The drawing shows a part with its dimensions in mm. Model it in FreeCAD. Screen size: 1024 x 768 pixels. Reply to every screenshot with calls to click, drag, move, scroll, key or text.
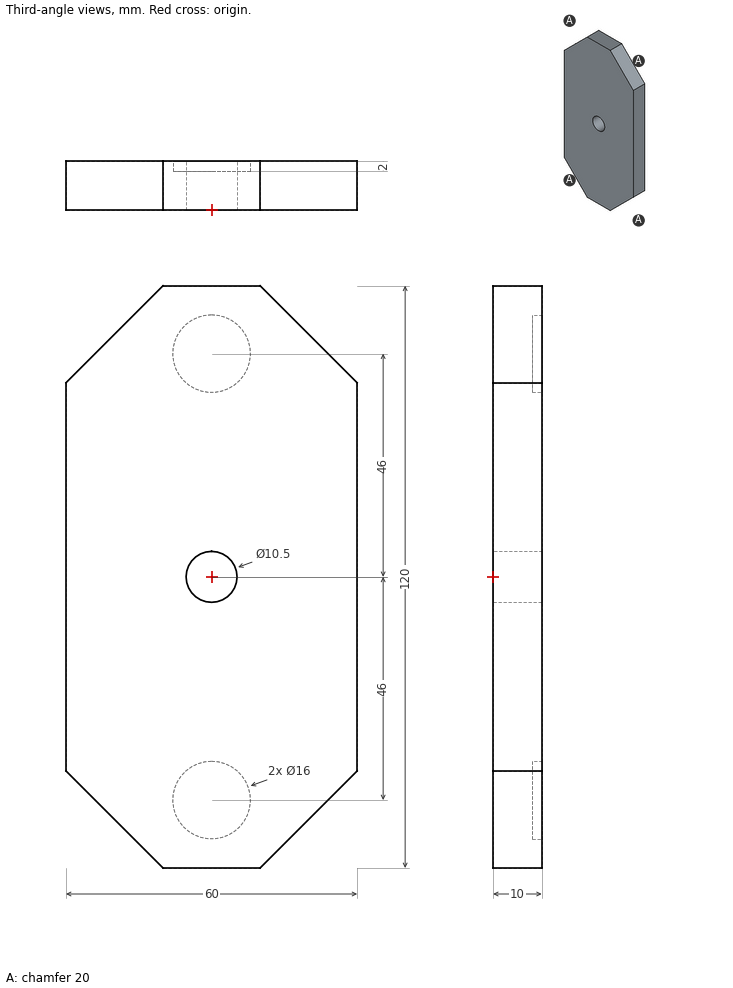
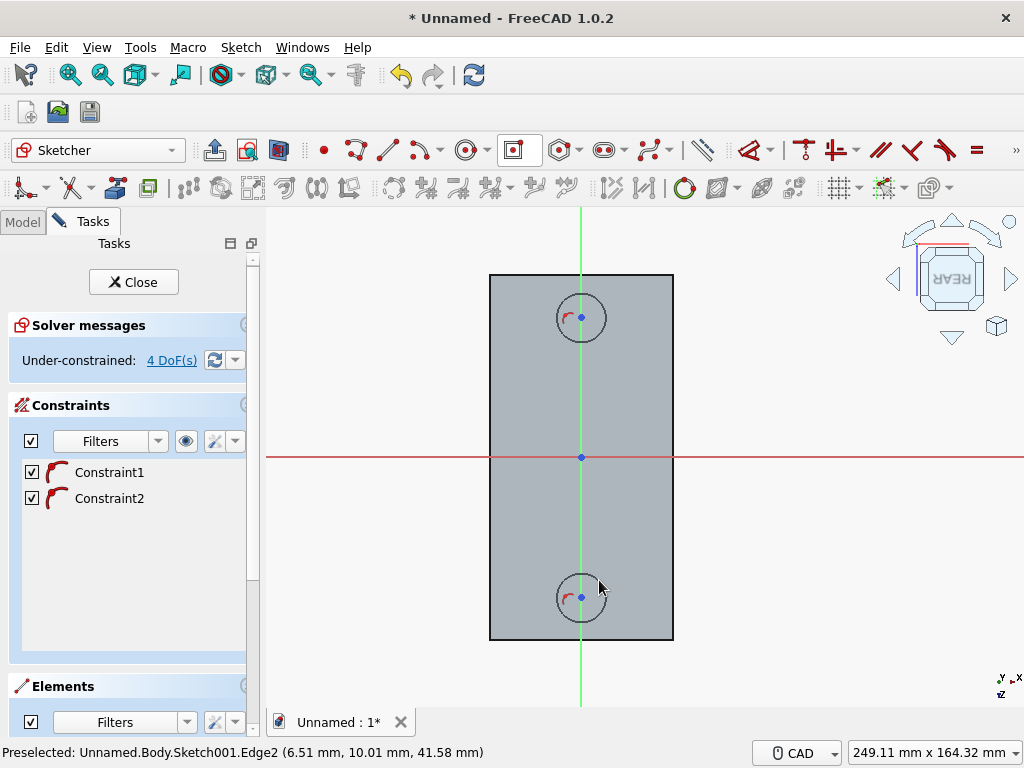
click(599, 301)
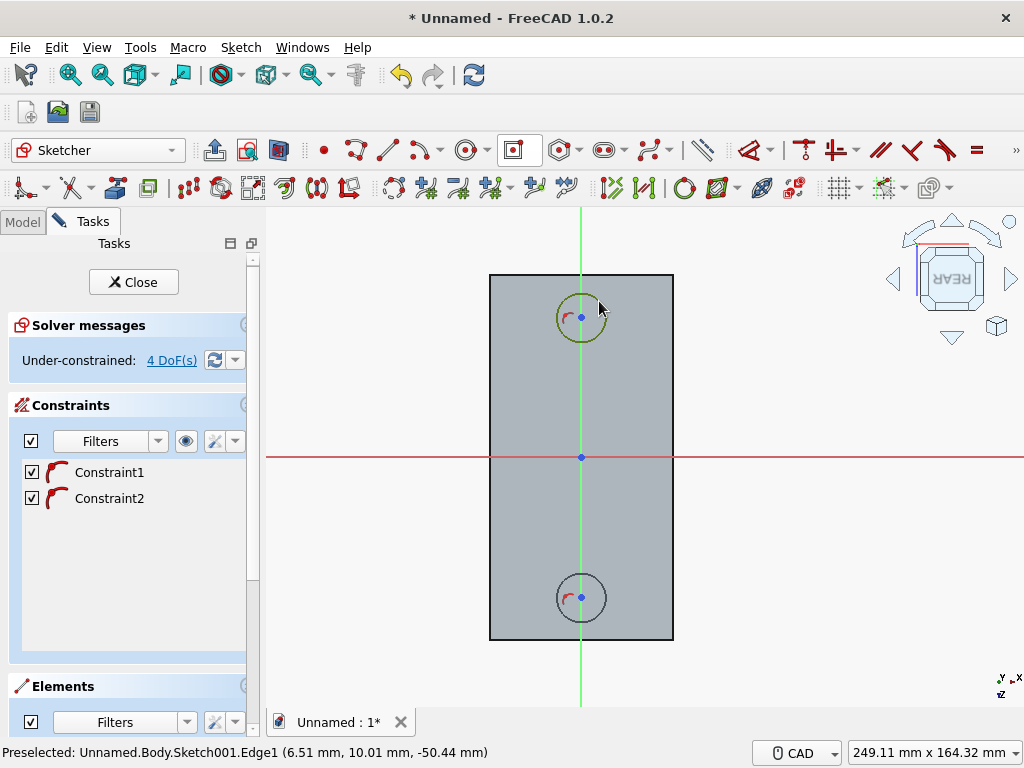
click(599, 581)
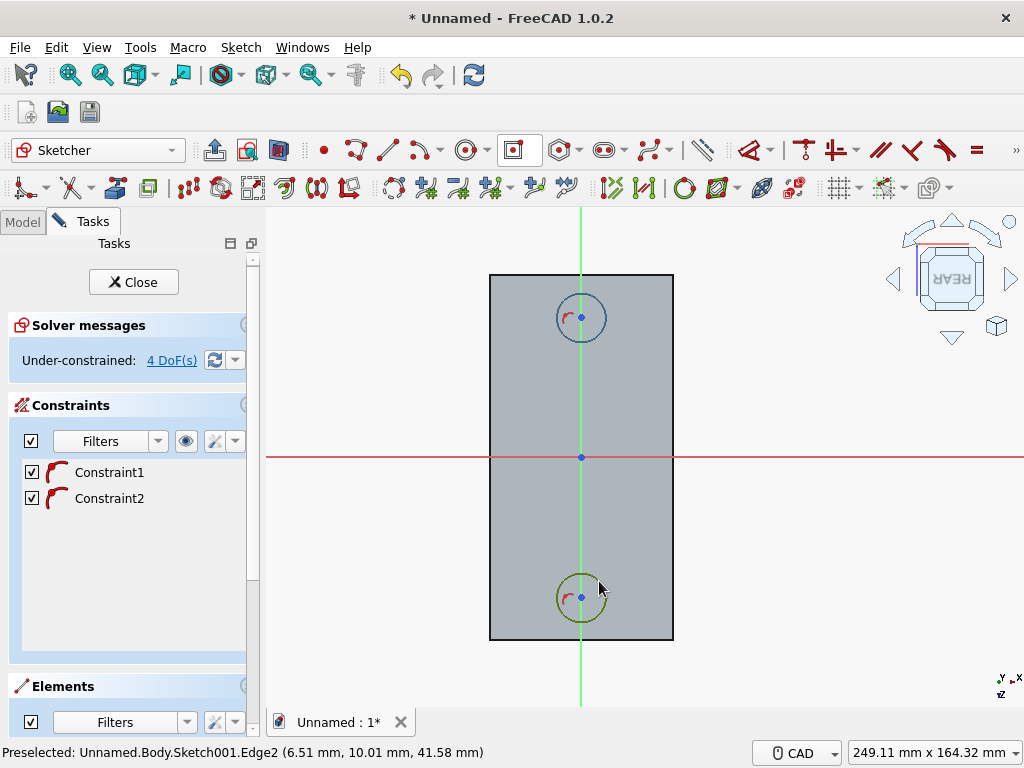
click(978, 150)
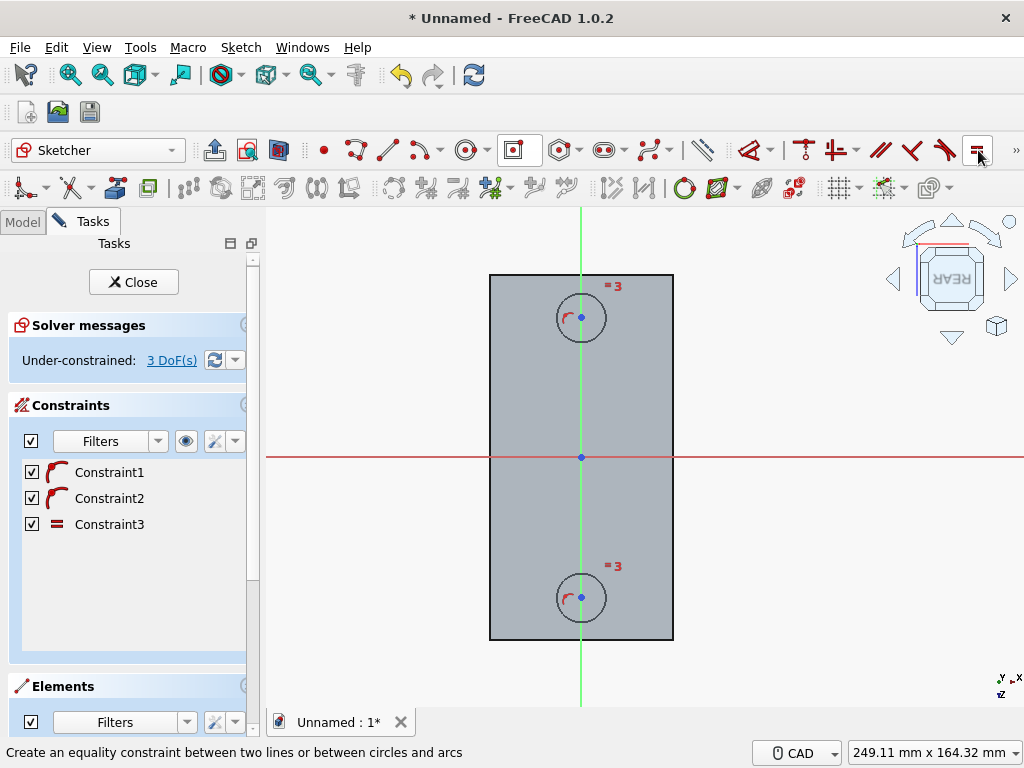
click(750, 150)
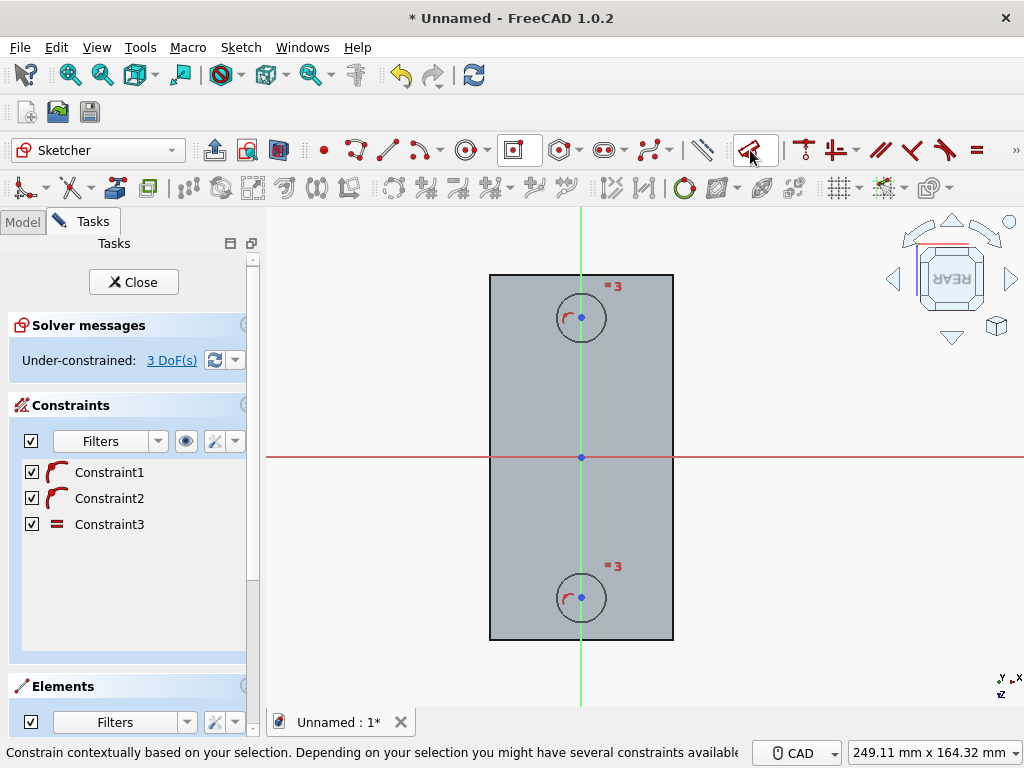
click(599, 301)
click(622, 279)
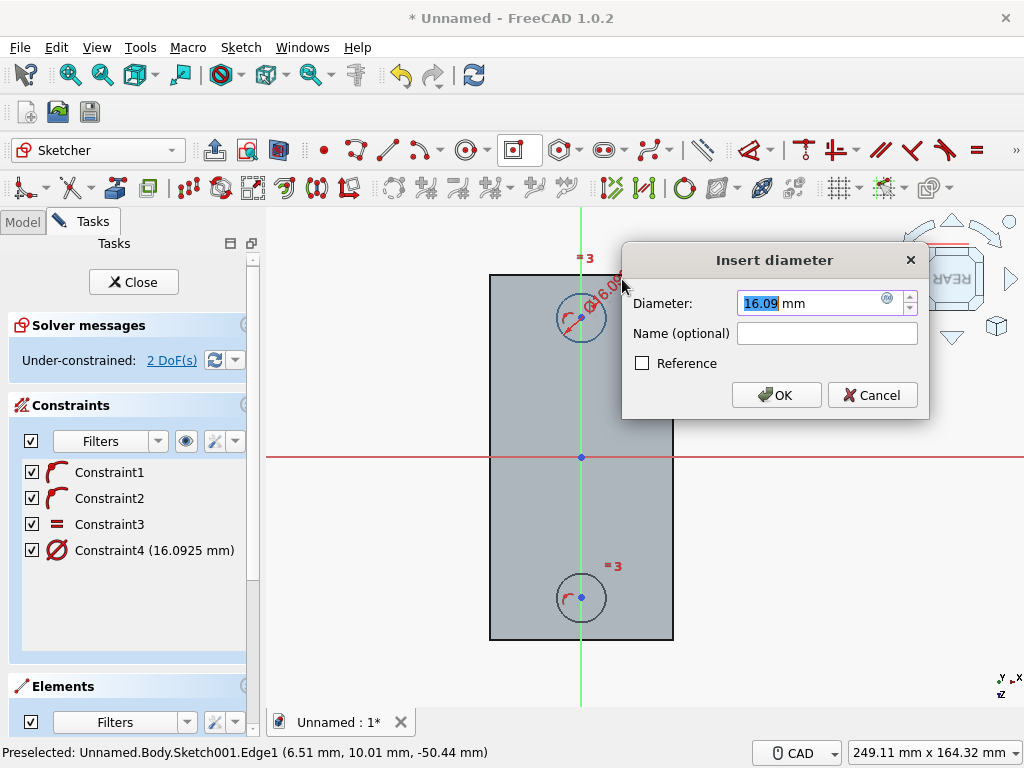
text(16)
key(Return)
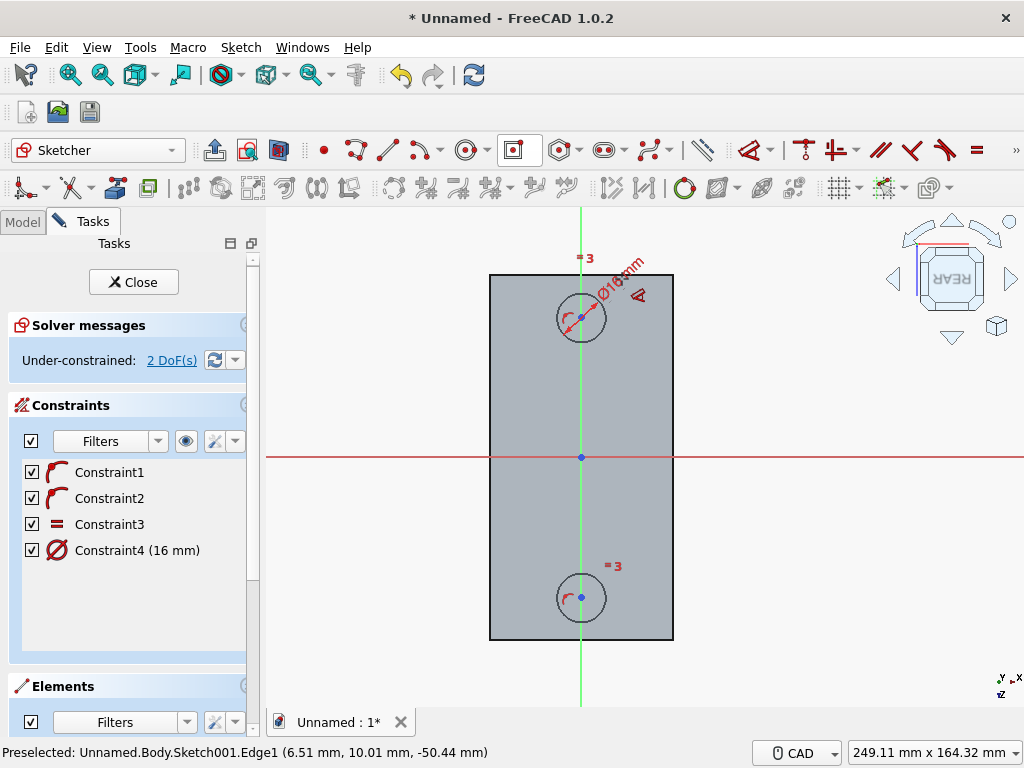
click(581, 318)
click(615, 388)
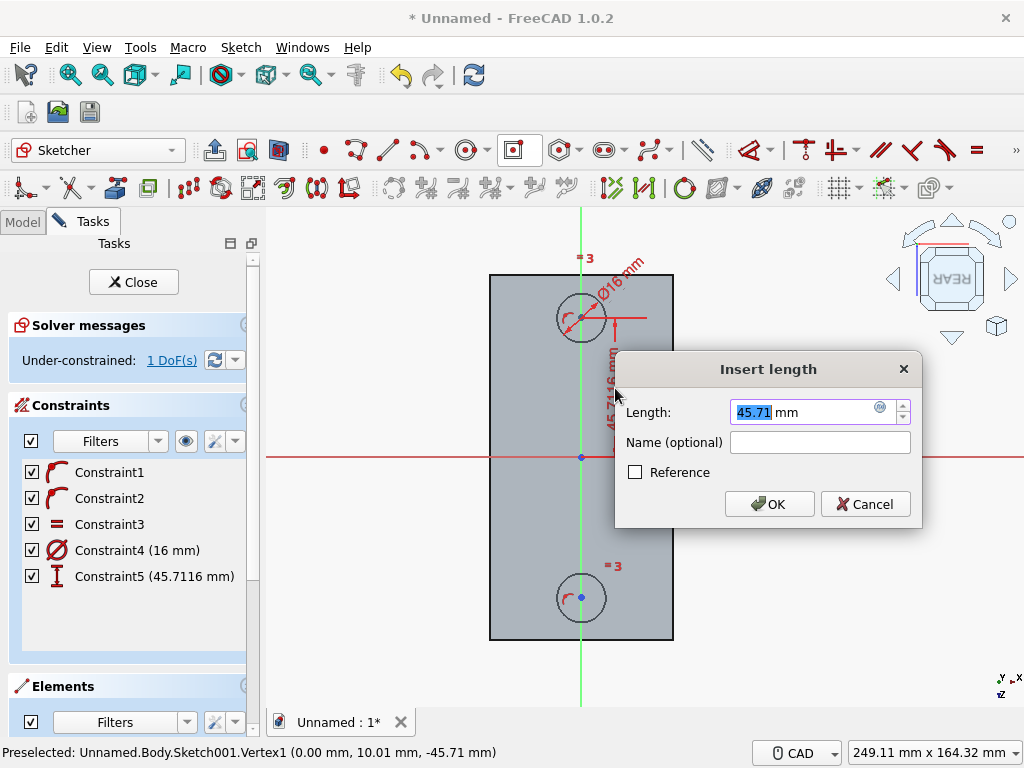
text(46)
key(Return)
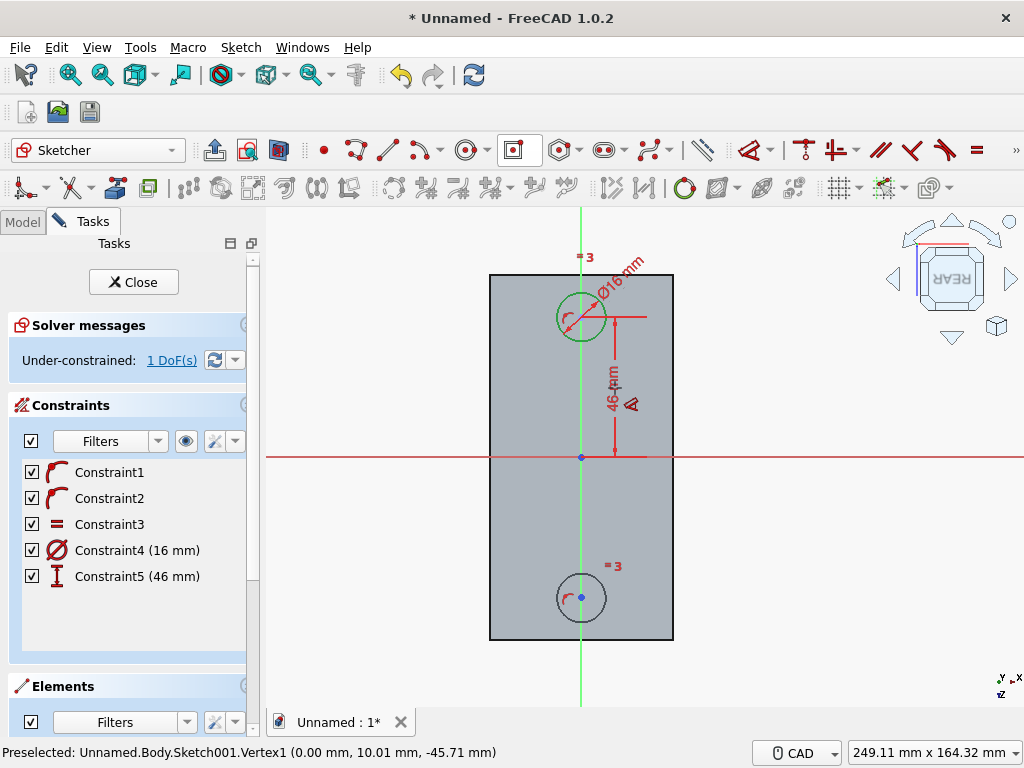
click(581, 598)
click(615, 528)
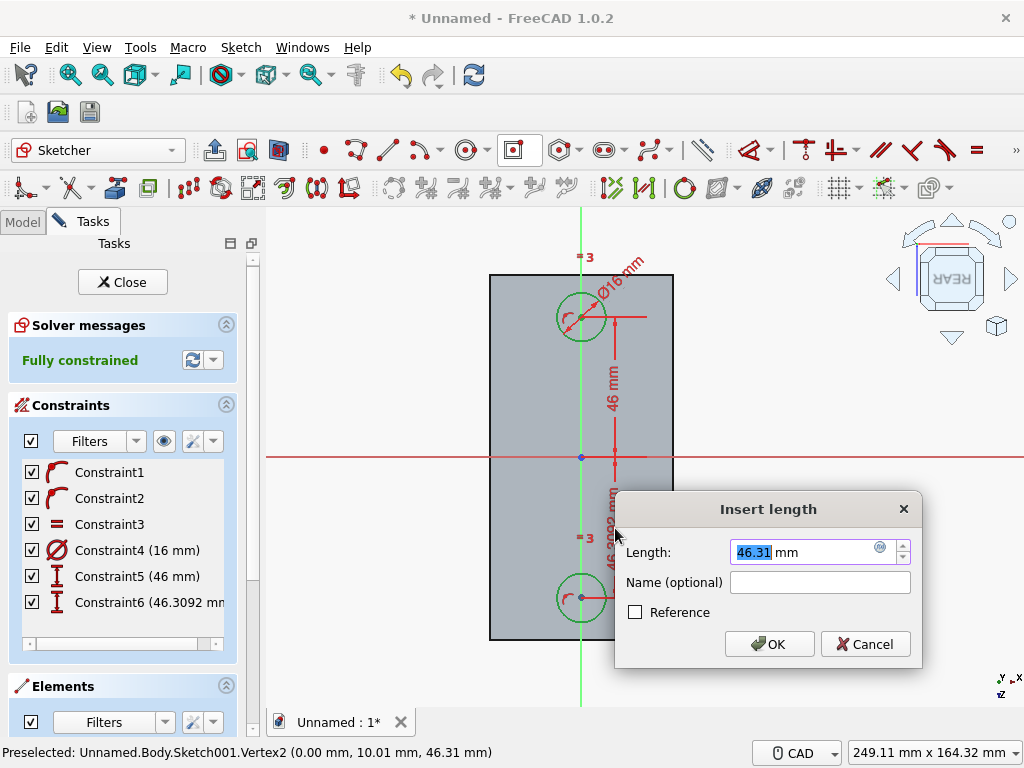
text(46)
key(Return)
key(Escape)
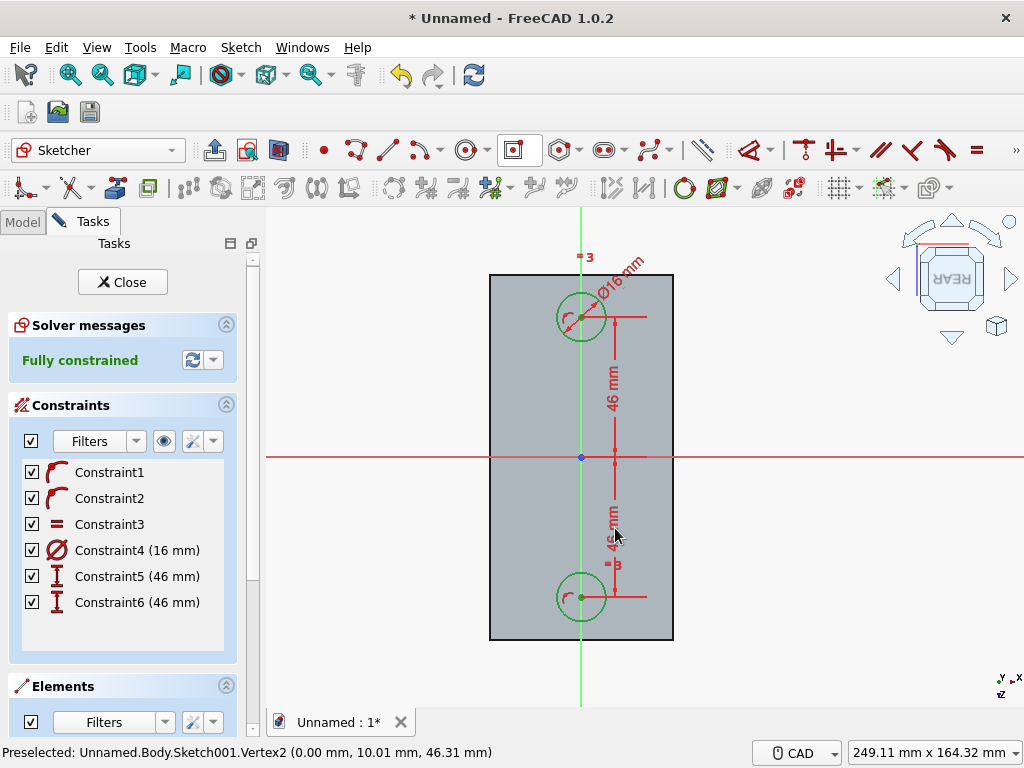
click(123, 282)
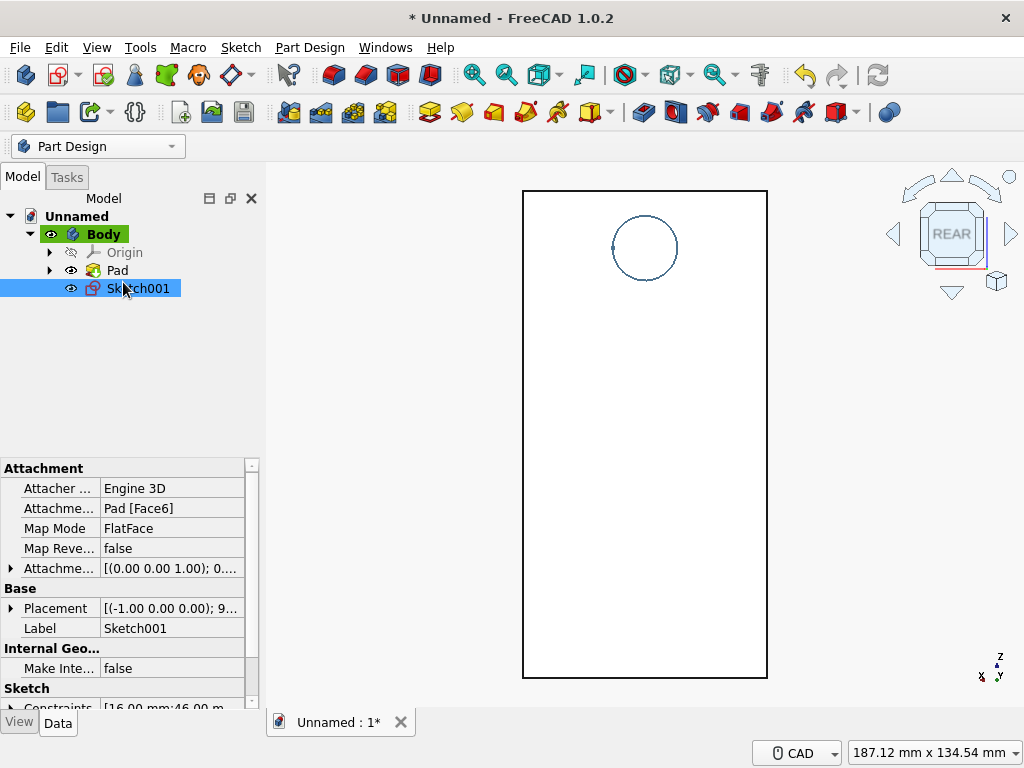
click(644, 112)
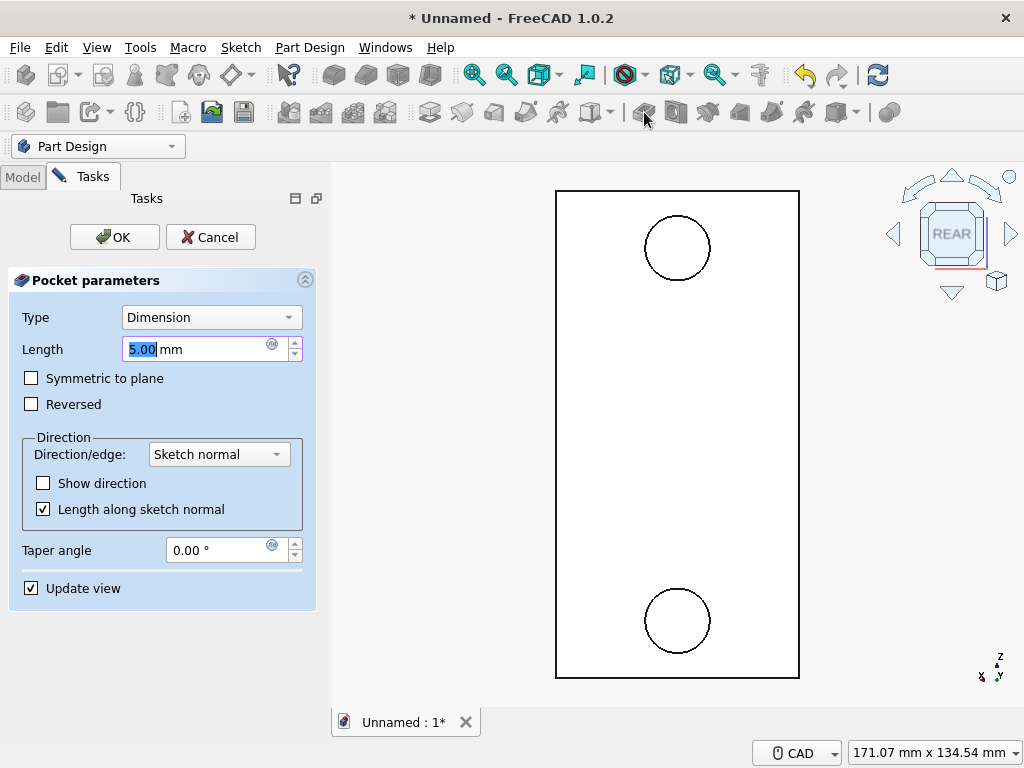
text(2)
key(Tab)